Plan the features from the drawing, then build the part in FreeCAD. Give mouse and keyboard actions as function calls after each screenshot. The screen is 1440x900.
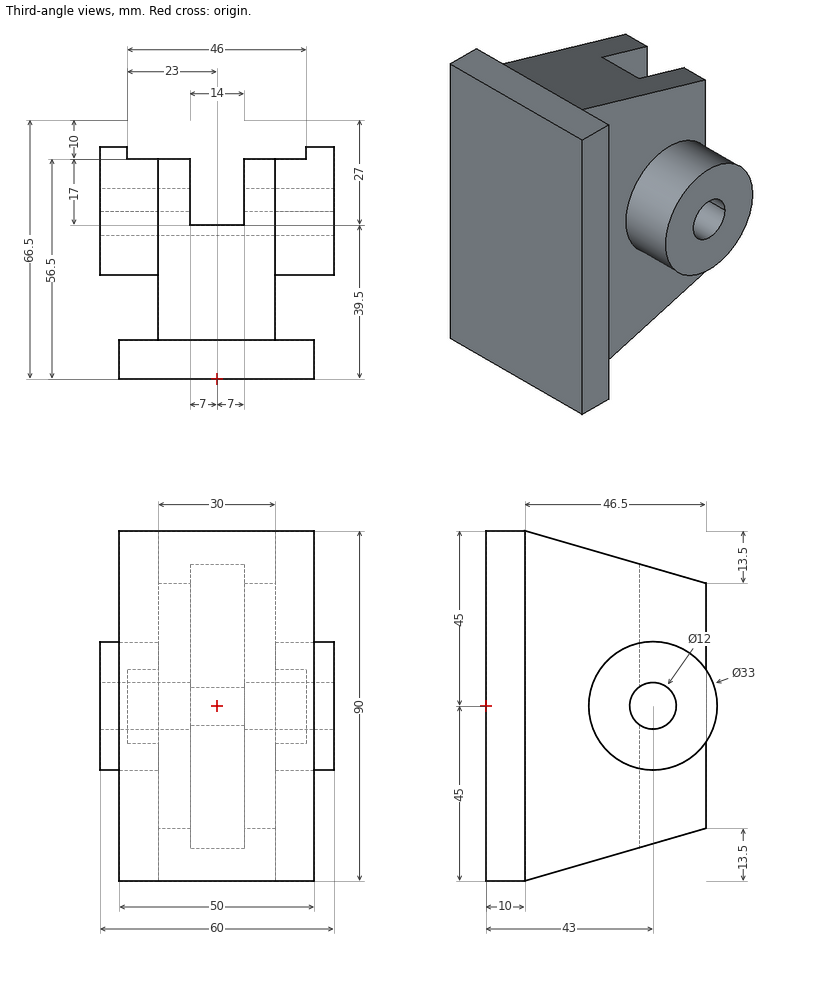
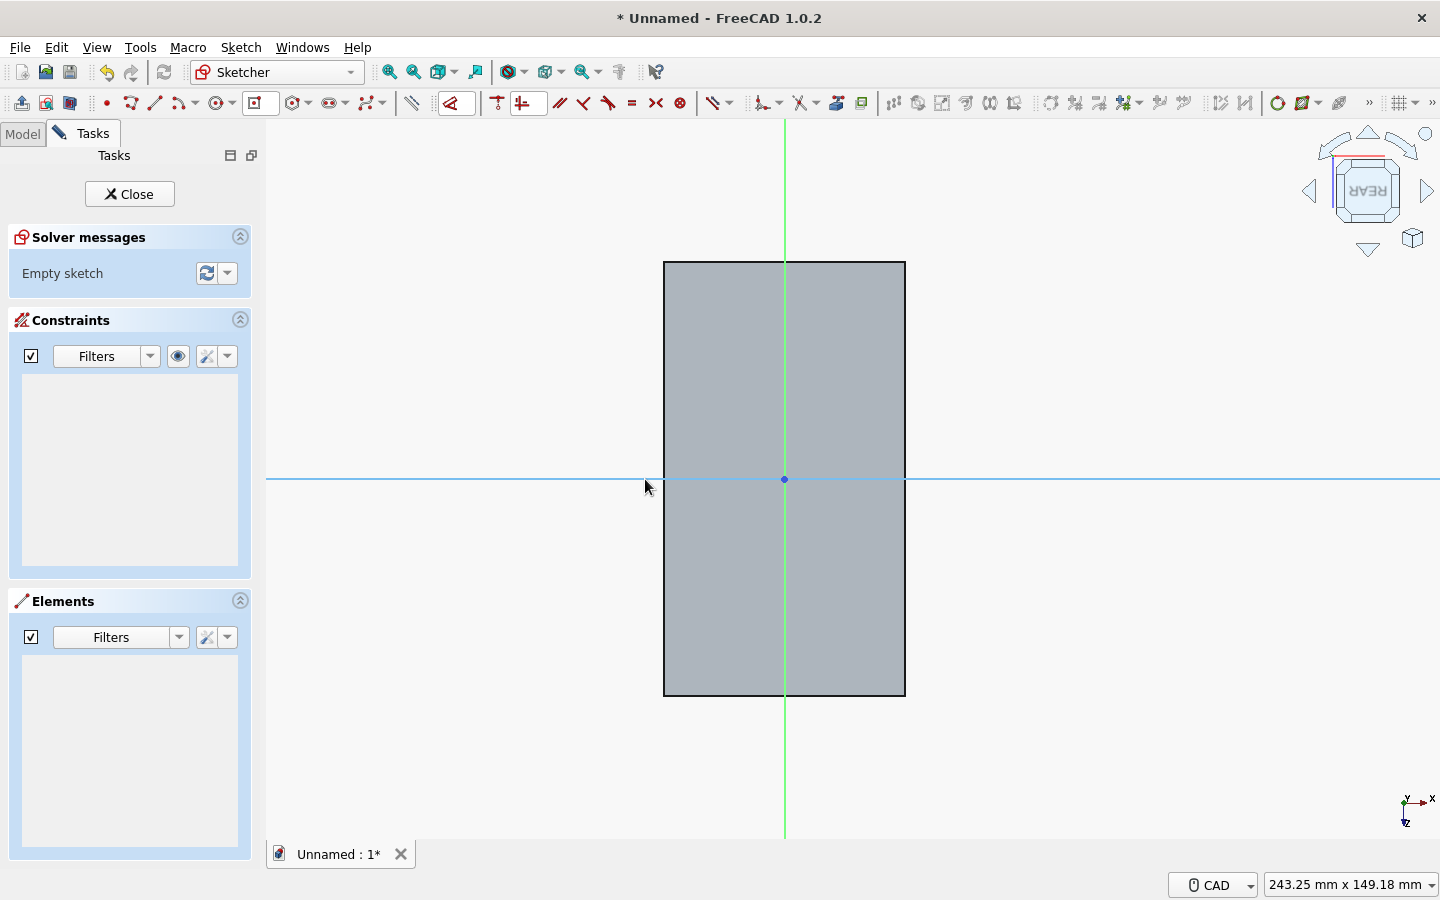
click(254, 104)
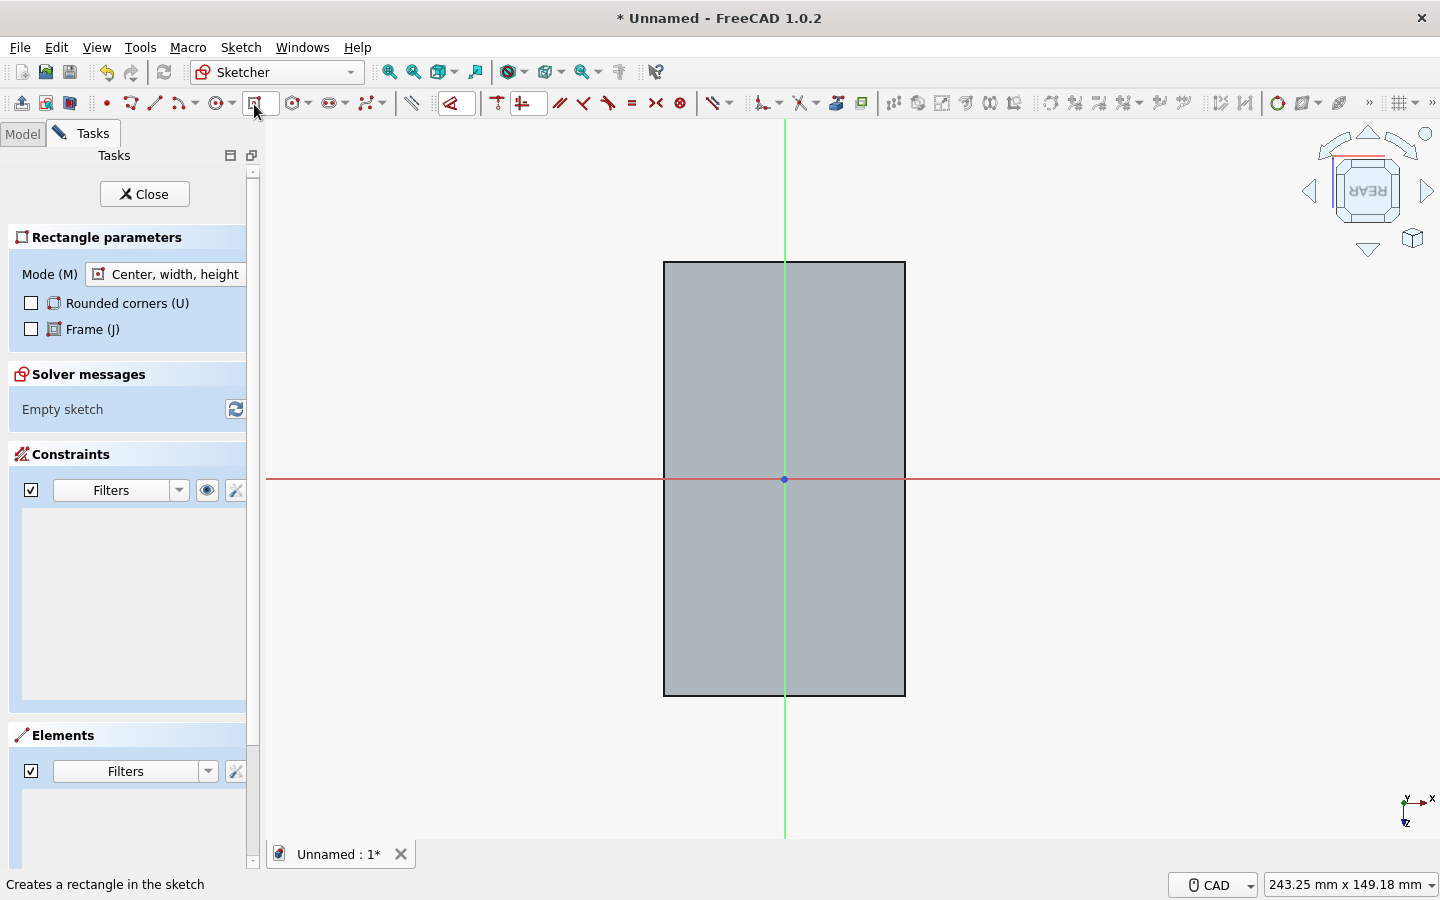
click(785, 479)
click(857, 262)
key(Escape)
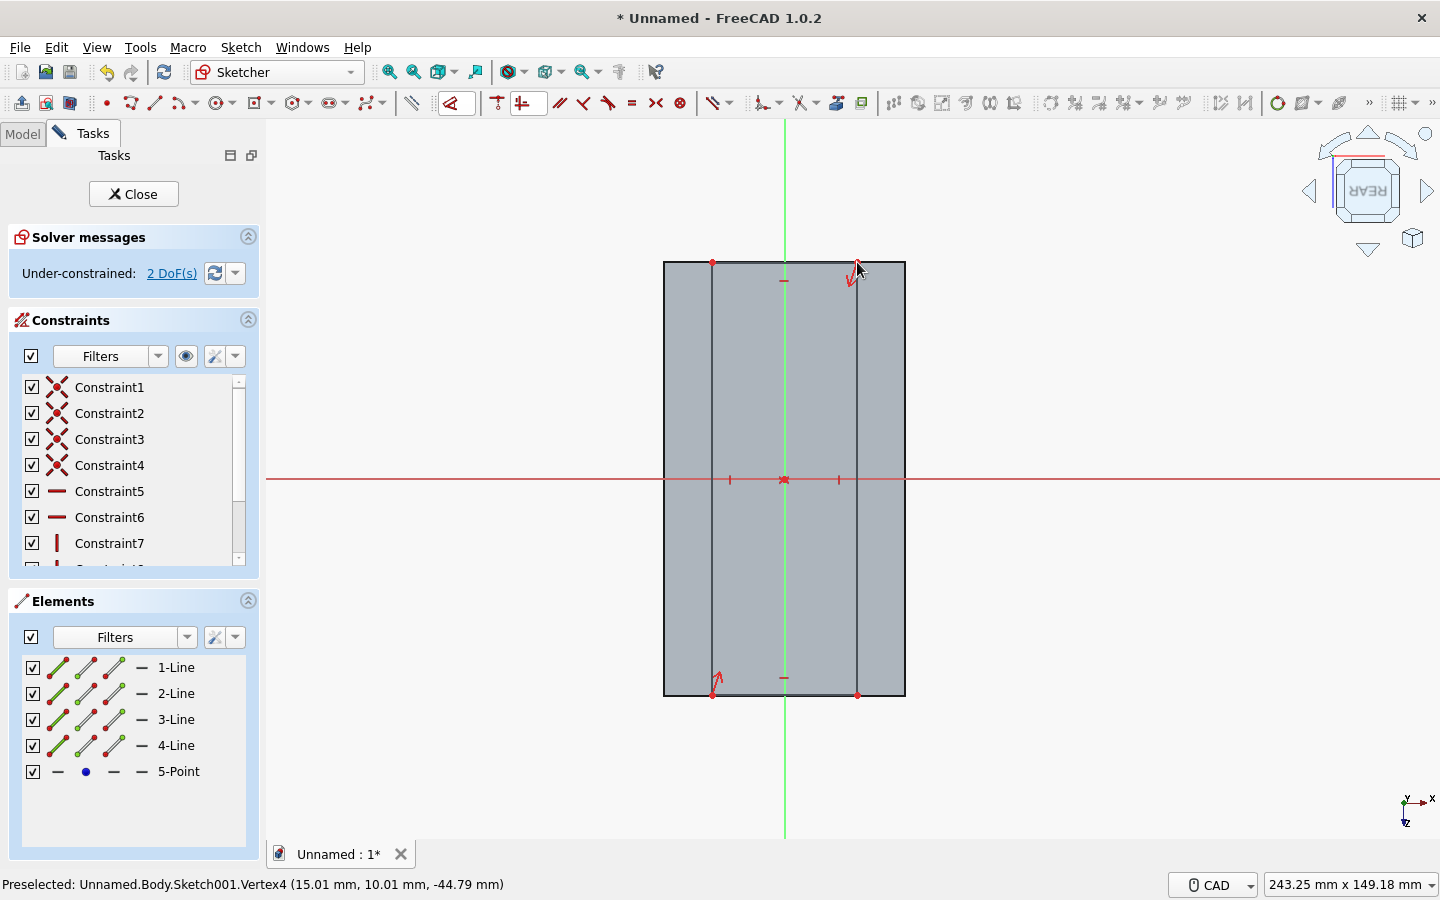
click(756, 695)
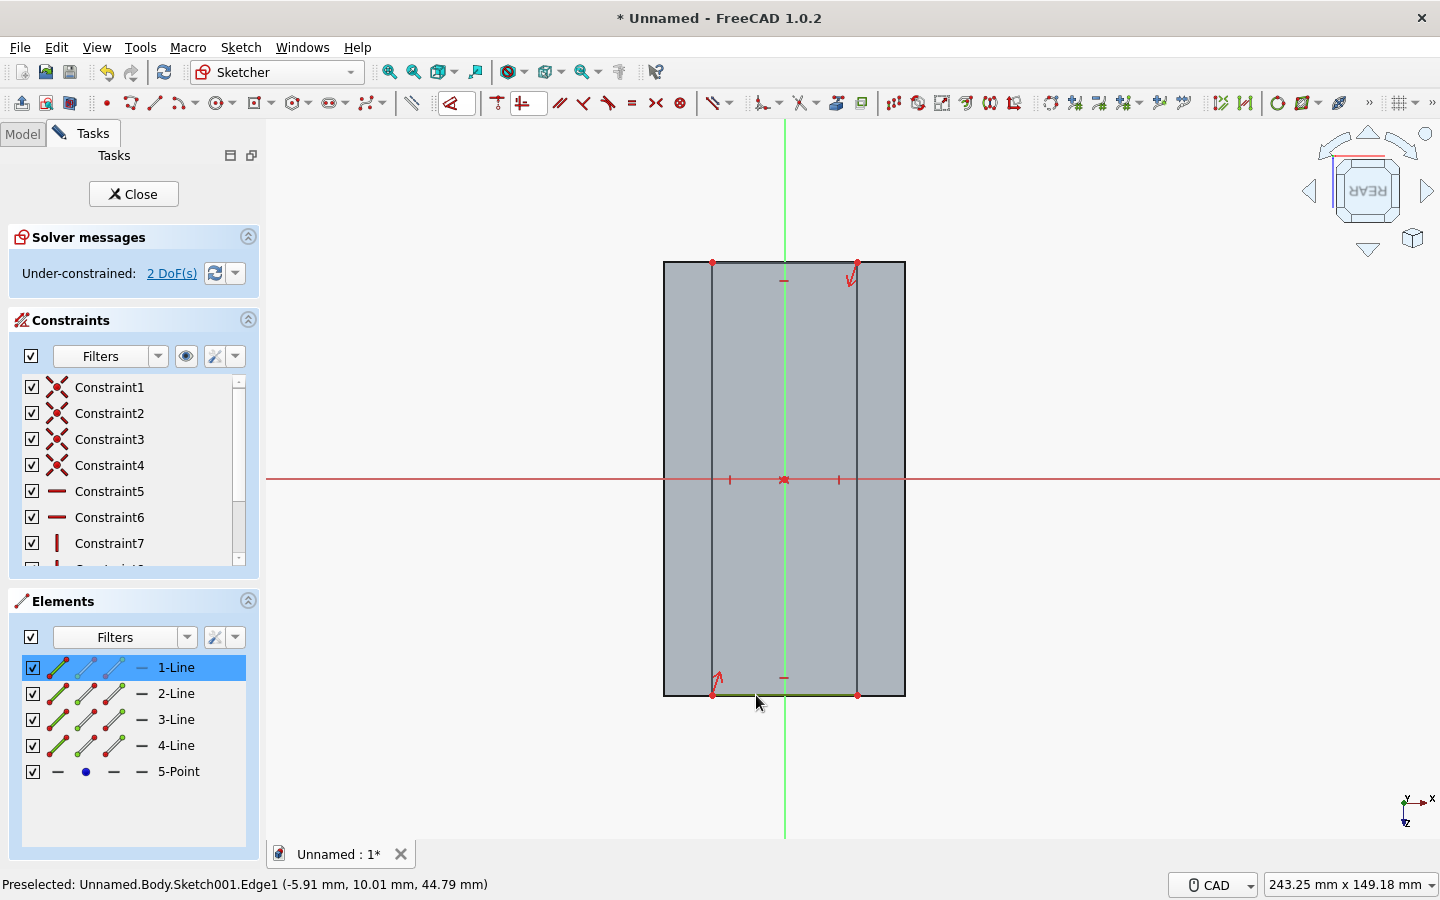
click(470, 104)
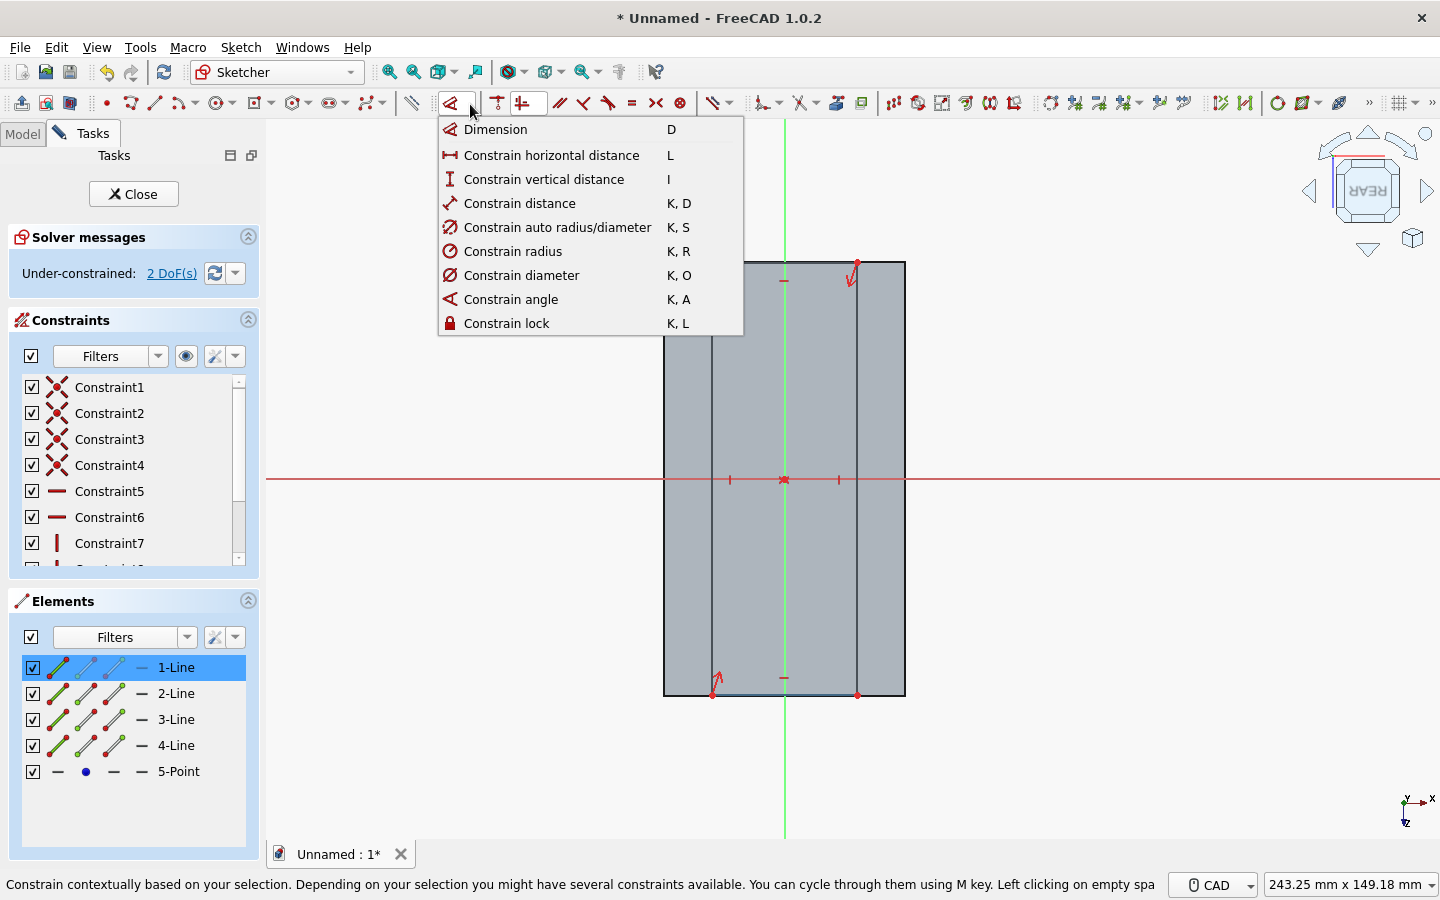
click(591, 155)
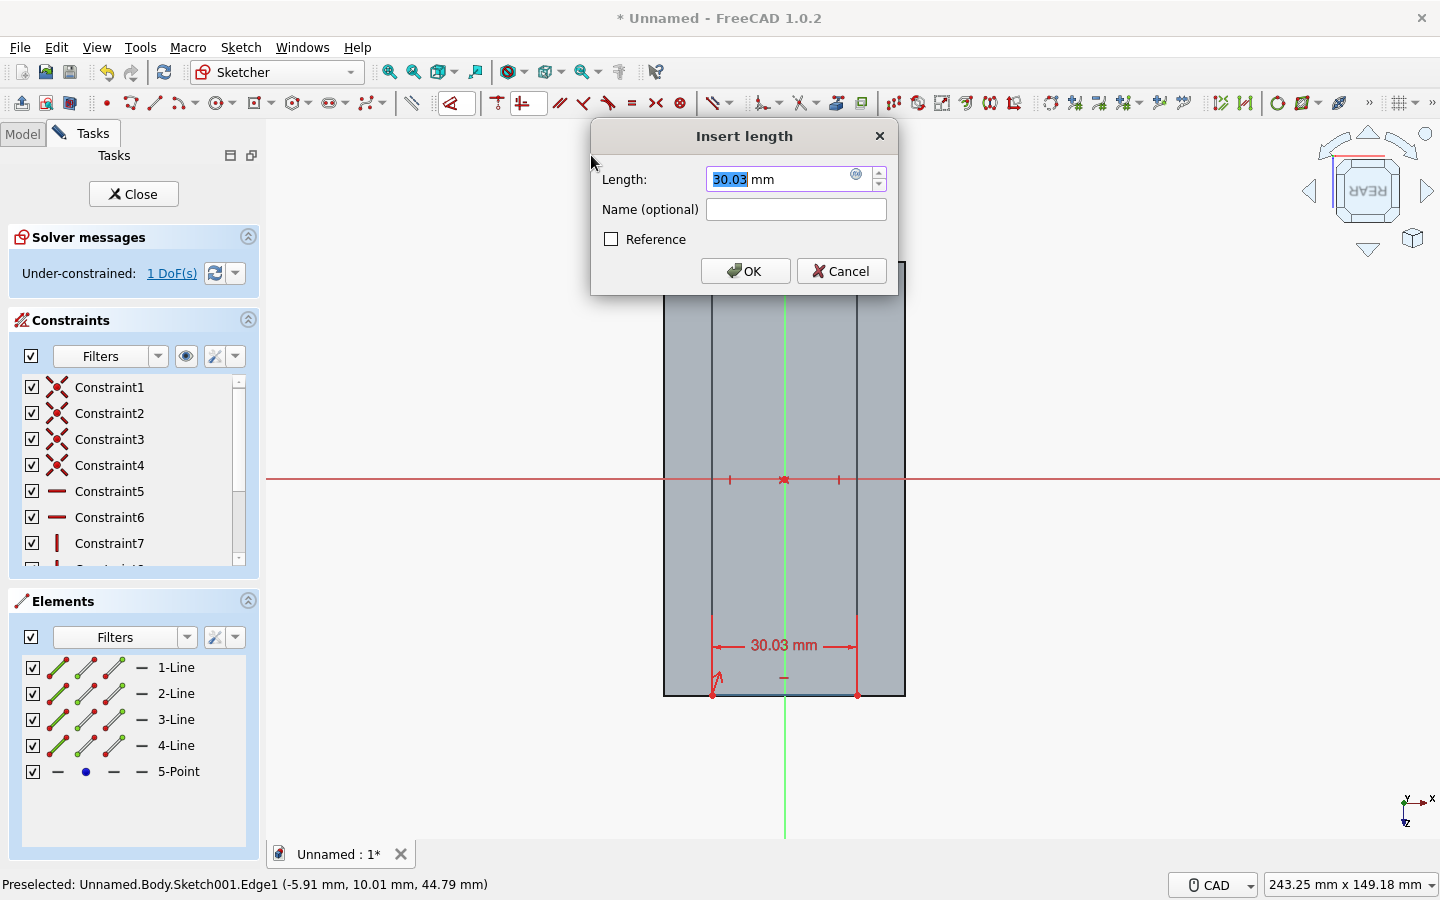
text(30)
key(Return)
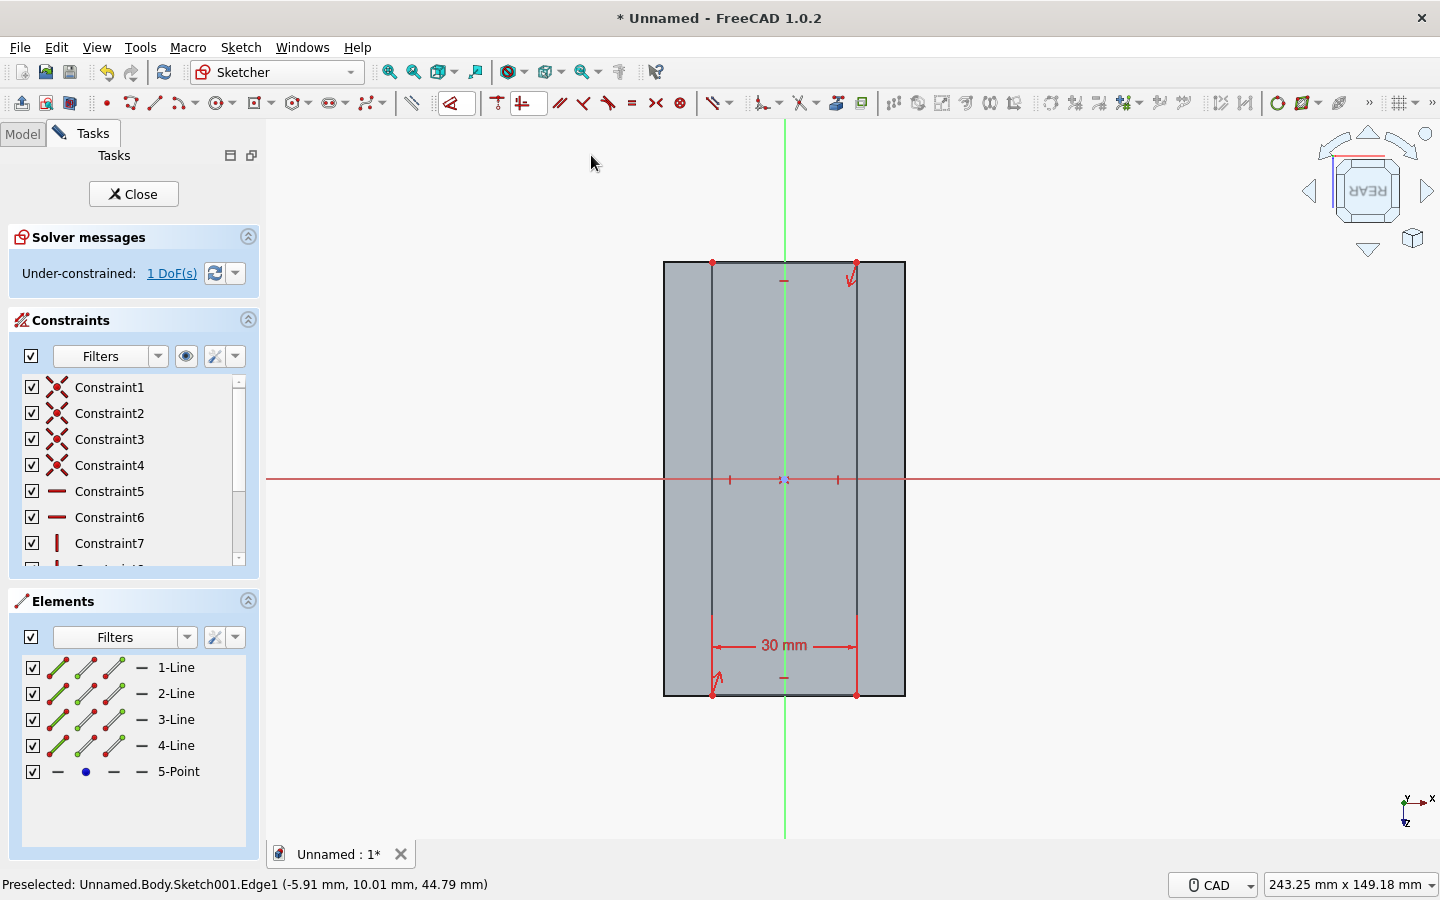
click(857, 566)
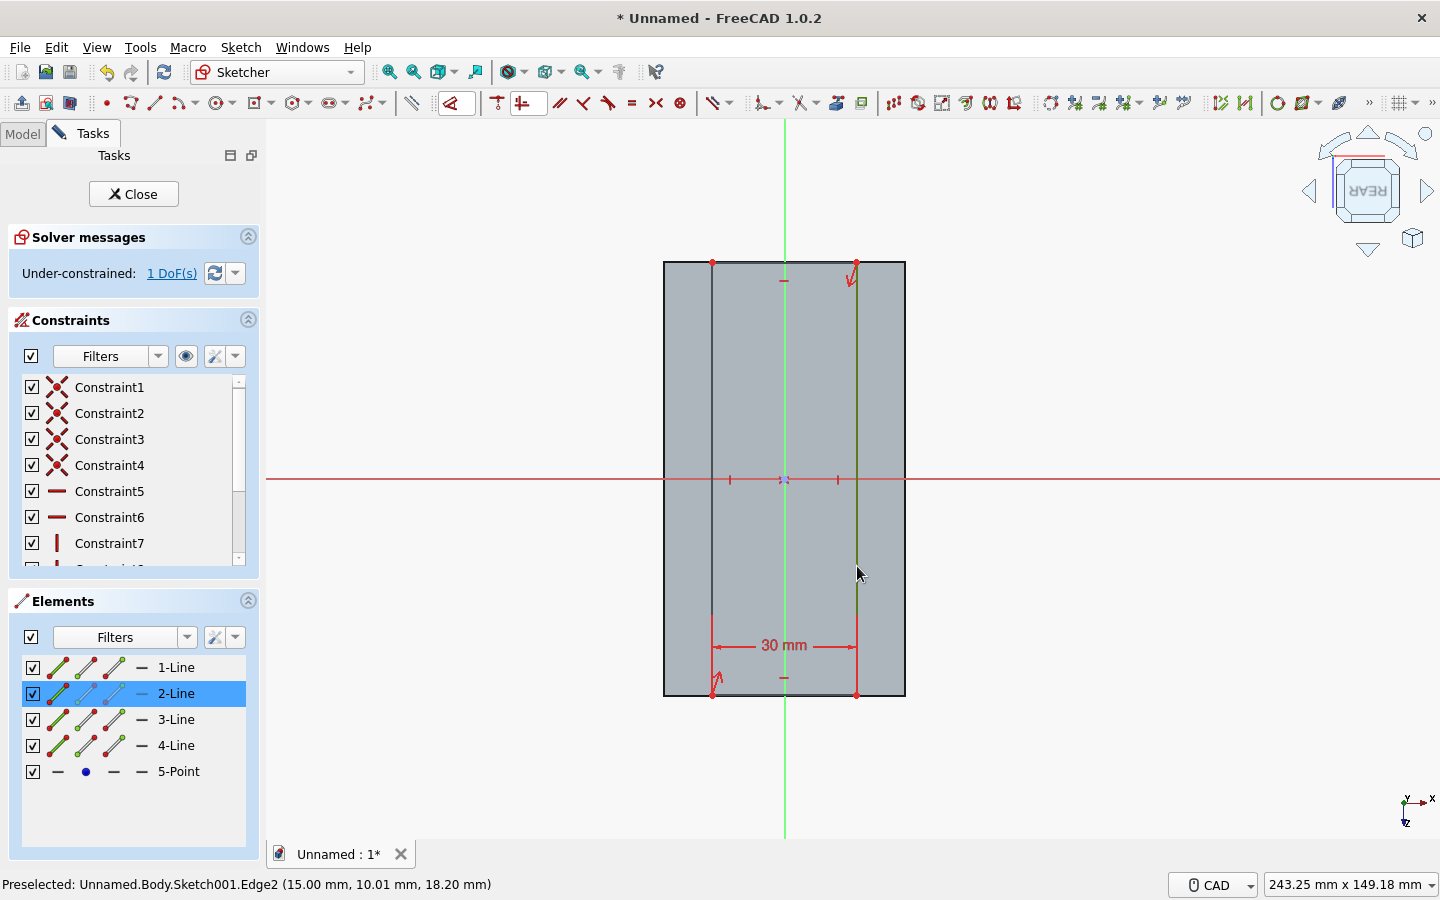
key(i)